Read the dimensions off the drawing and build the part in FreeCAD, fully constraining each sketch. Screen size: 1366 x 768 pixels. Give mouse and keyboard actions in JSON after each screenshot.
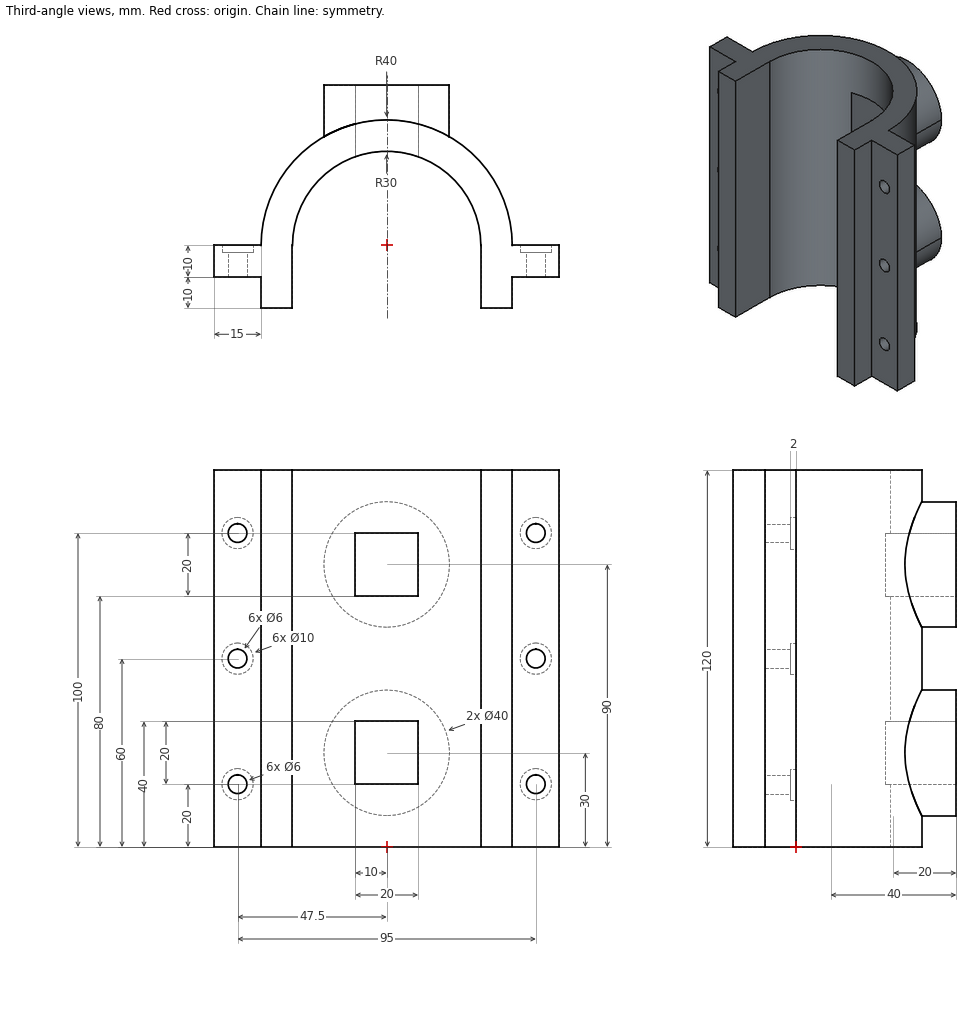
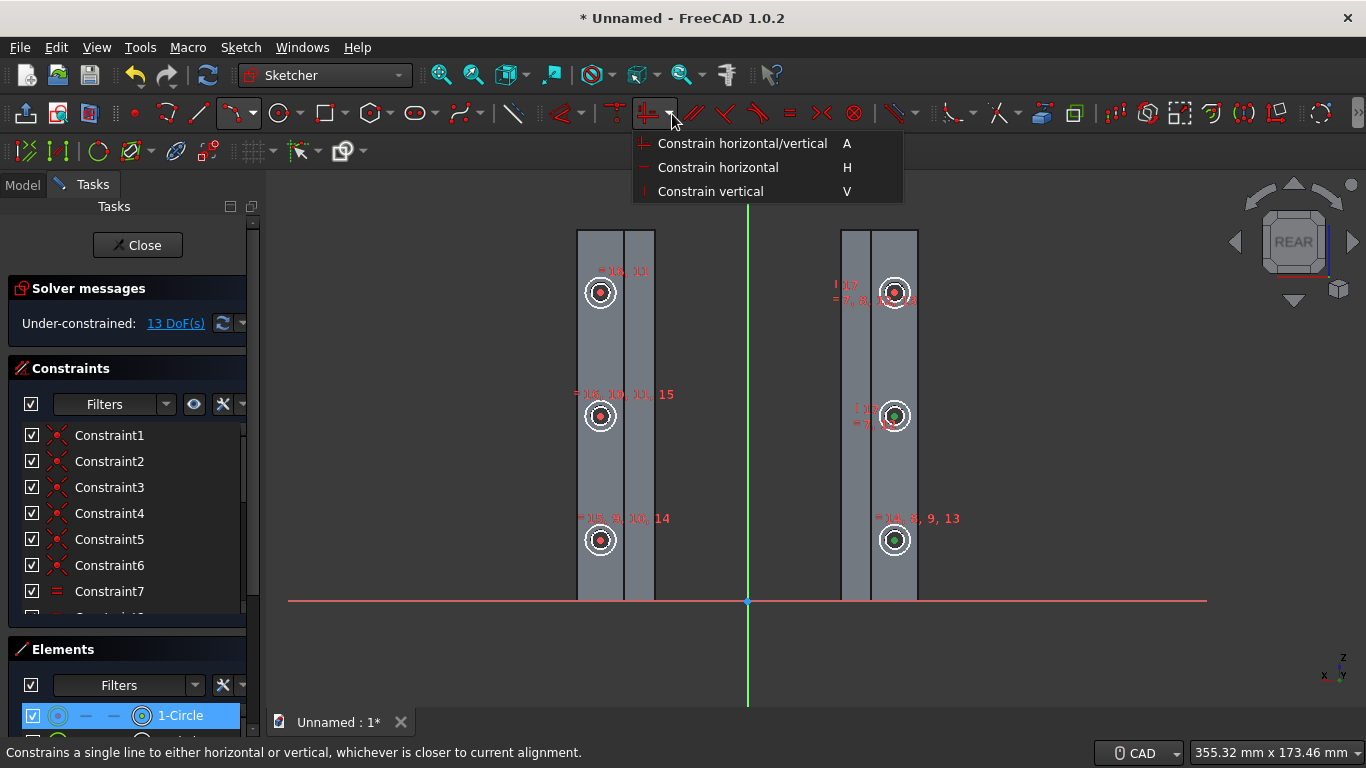
{"action": "left_click", "coordinate": [768, 191]}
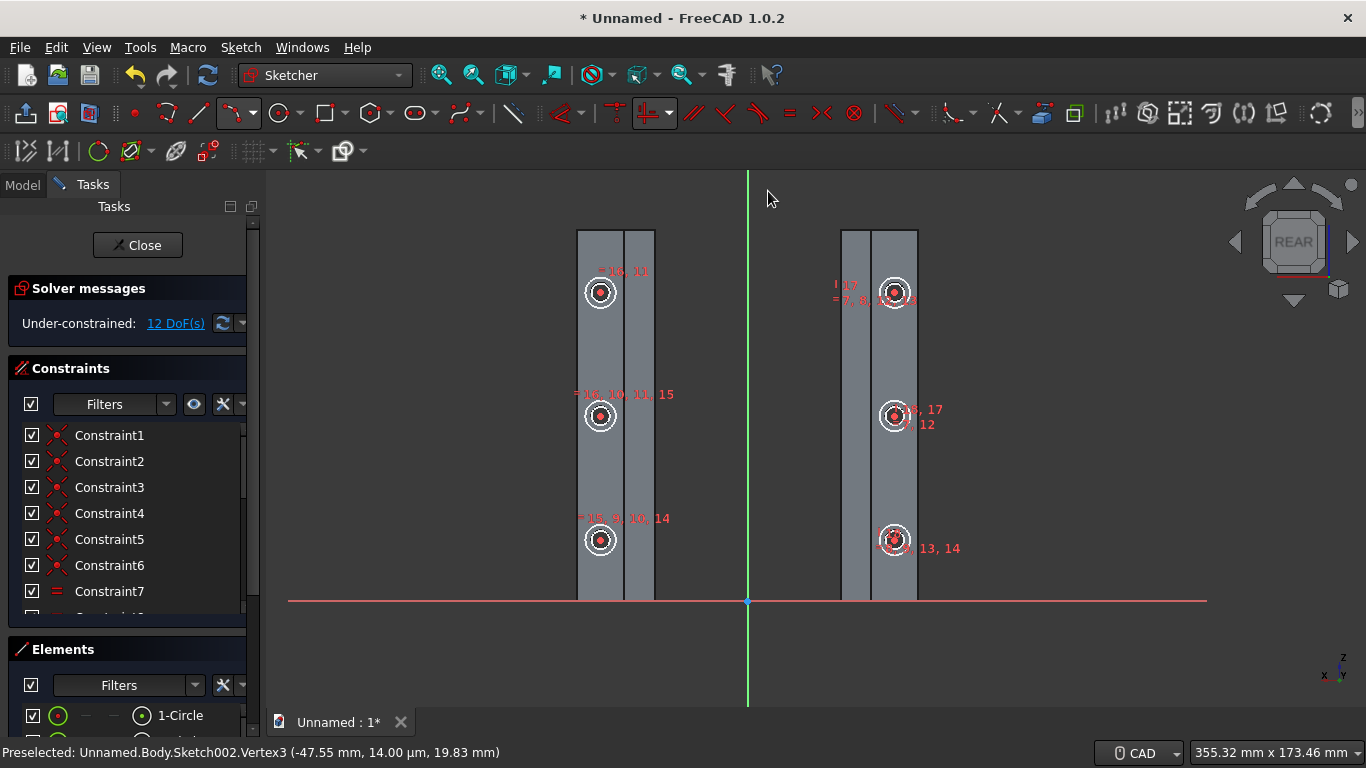
{"action": "scroll", "coordinate": [895, 540], "scroll_direction": "up", "scroll_amount": 4}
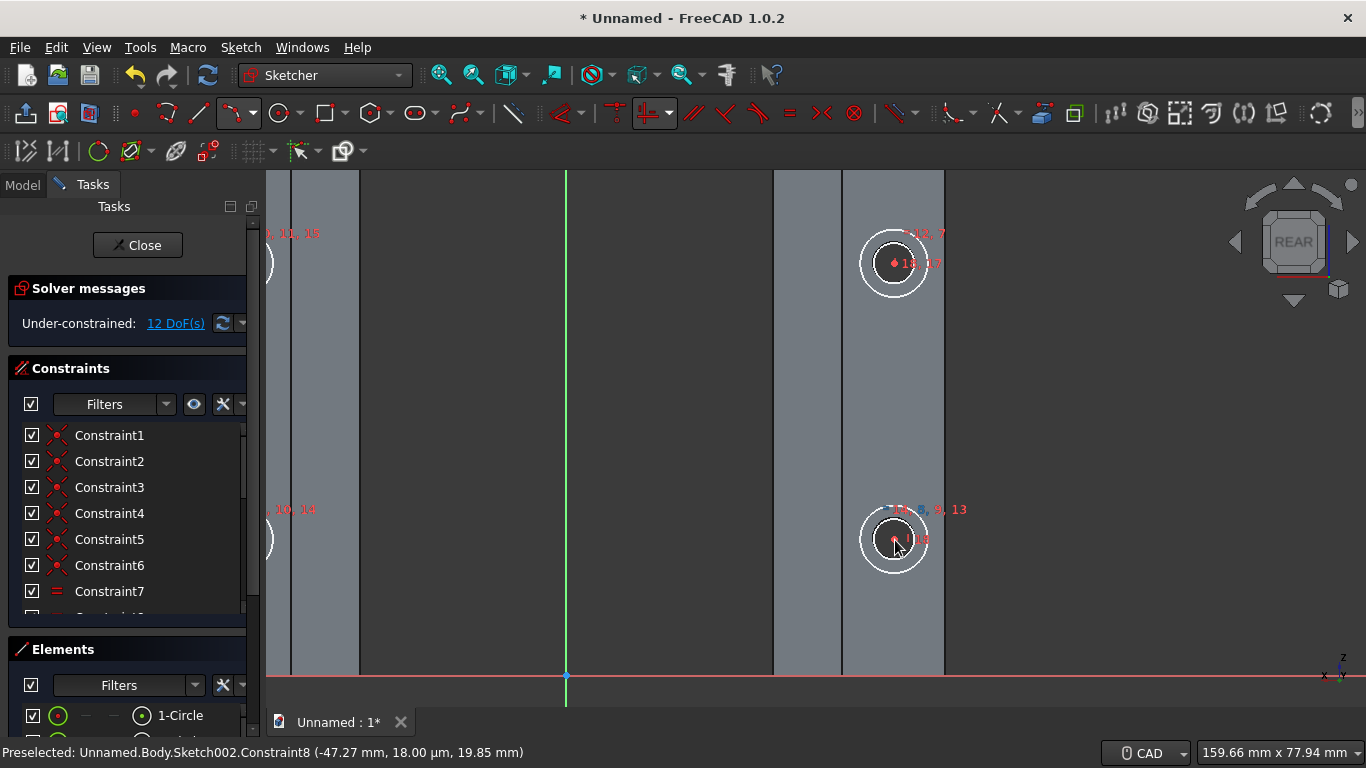
{"action": "left_click", "coordinate": [894, 539]}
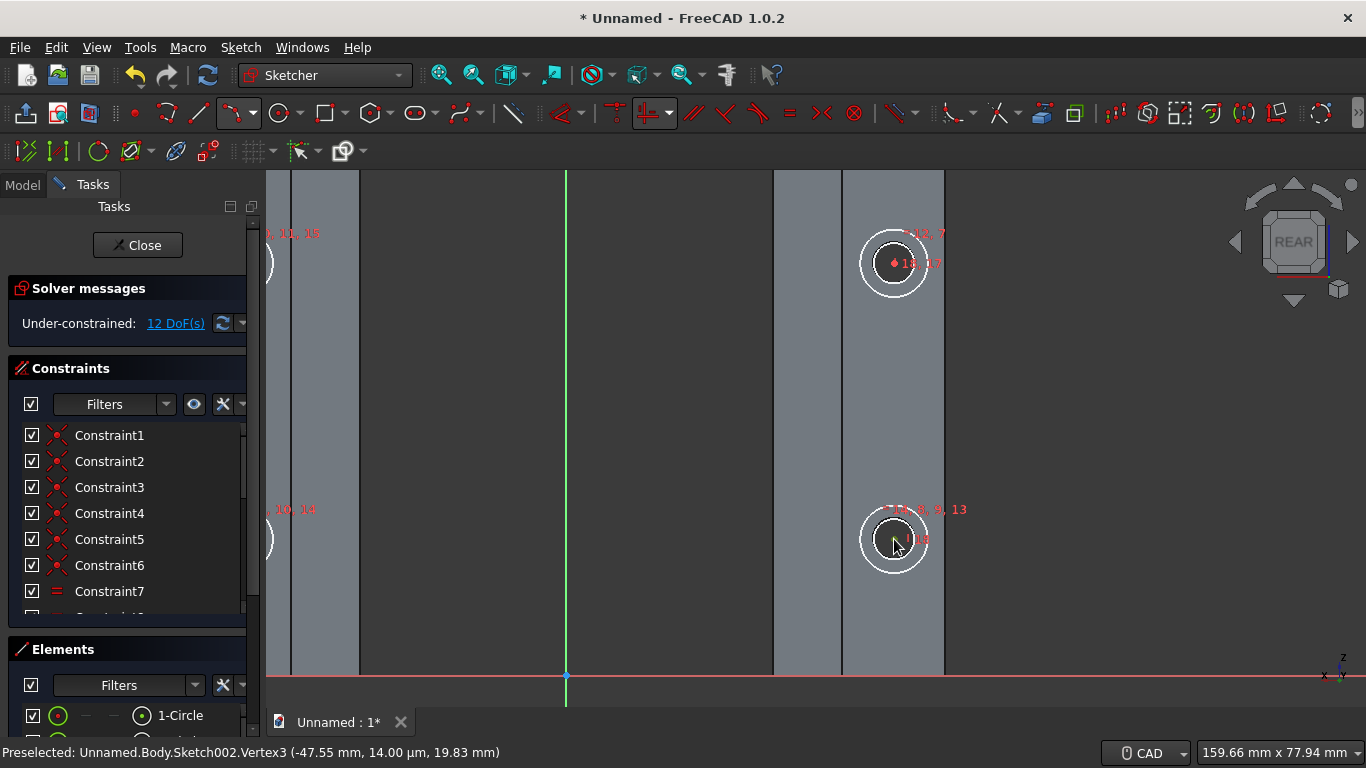
{"action": "scroll", "coordinate": [895, 540], "scroll_direction": "down", "scroll_amount": 4}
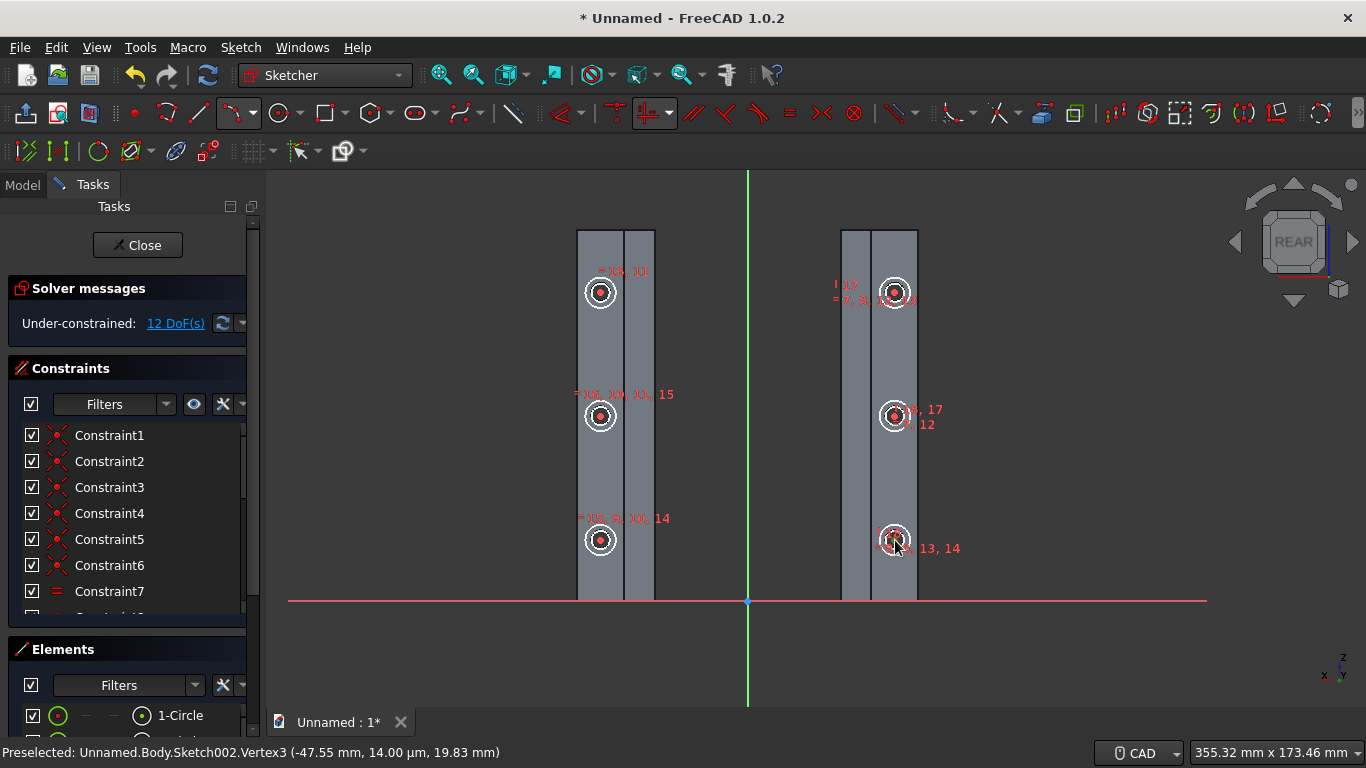
{"action": "left_click", "coordinate": [601, 540]}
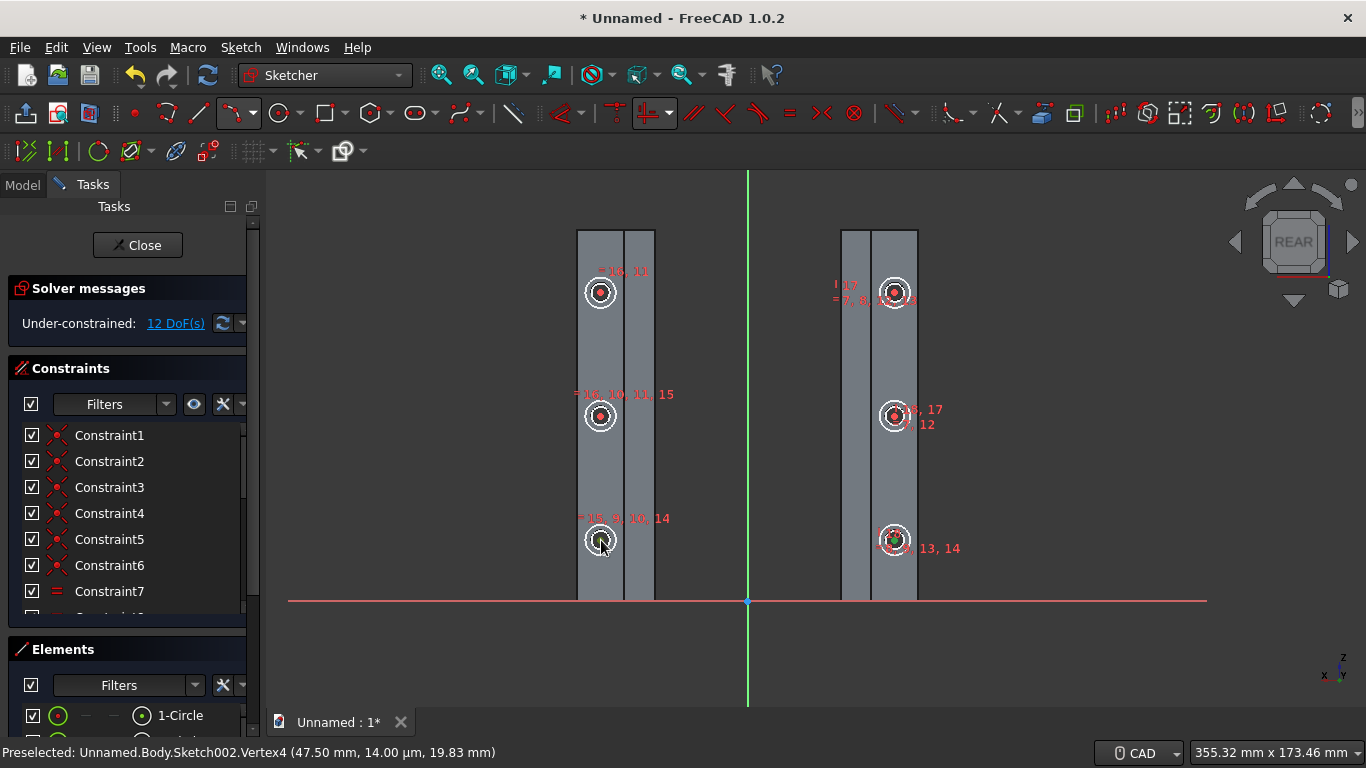
{"action": "left_click", "coordinate": [672, 114]}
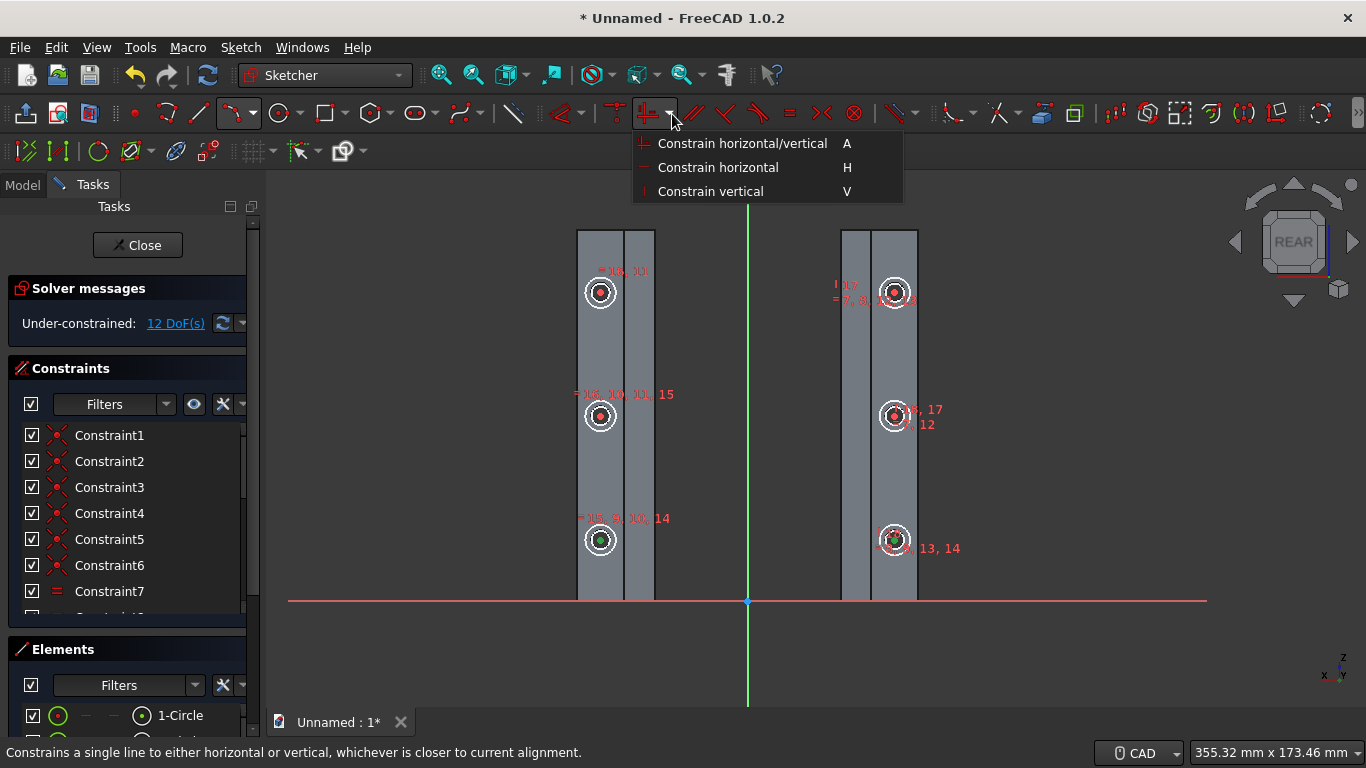
{"action": "left_click", "coordinate": [768, 167]}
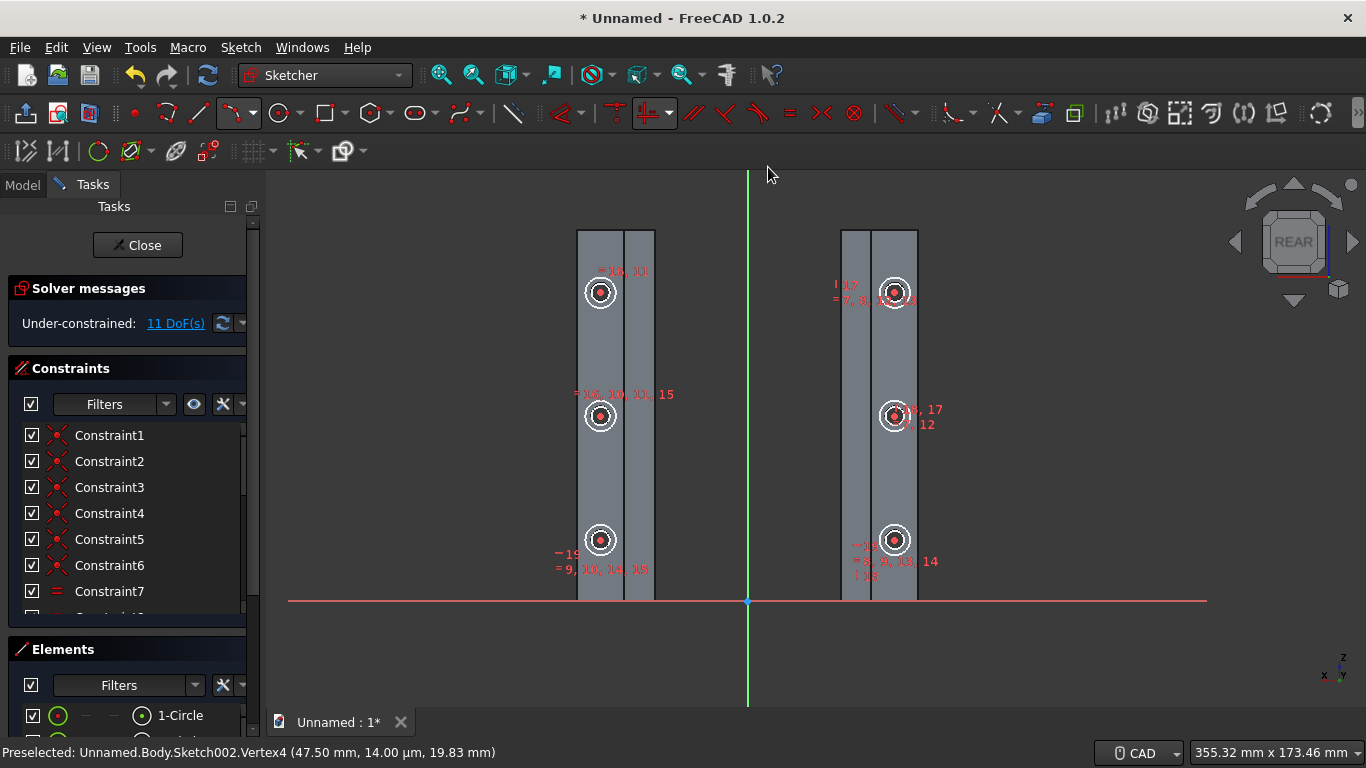
{"action": "left_click", "coordinate": [601, 540]}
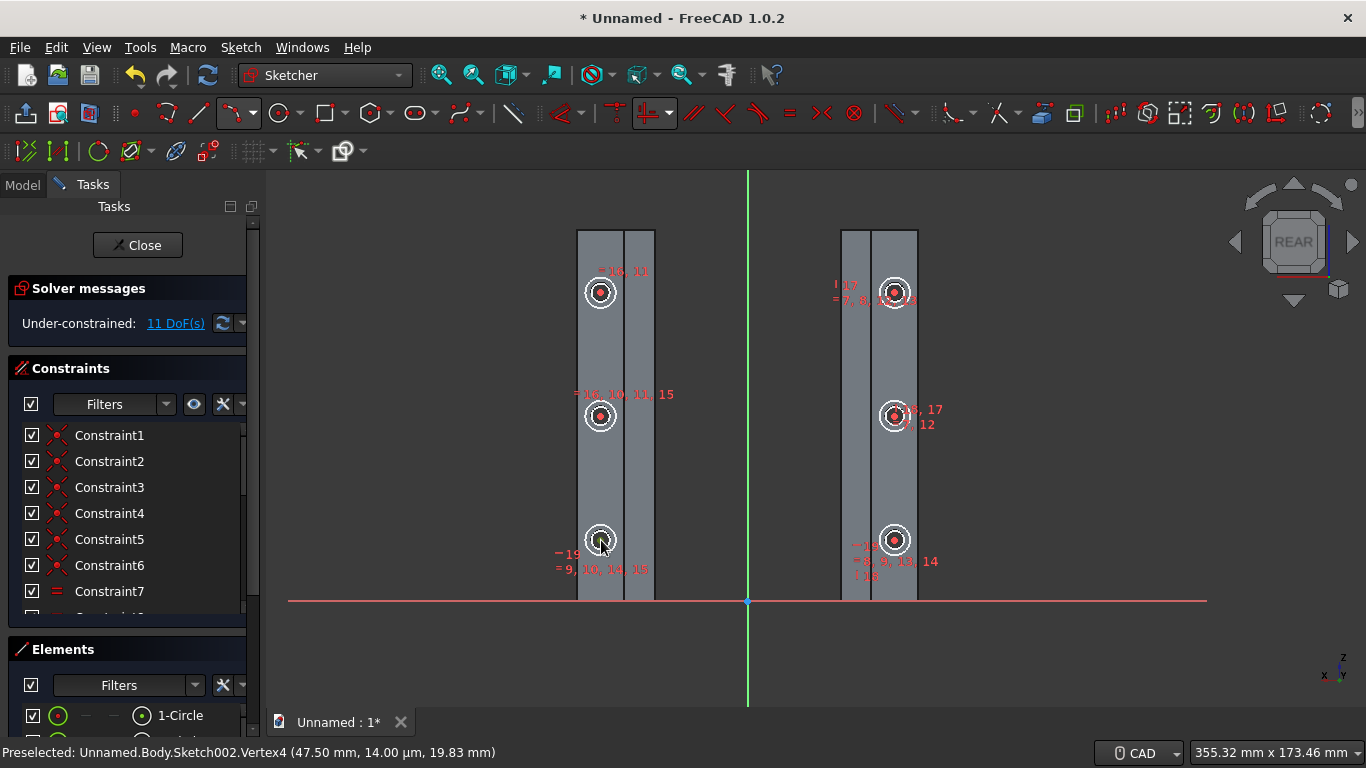
{"action": "left_click", "coordinate": [601, 416]}